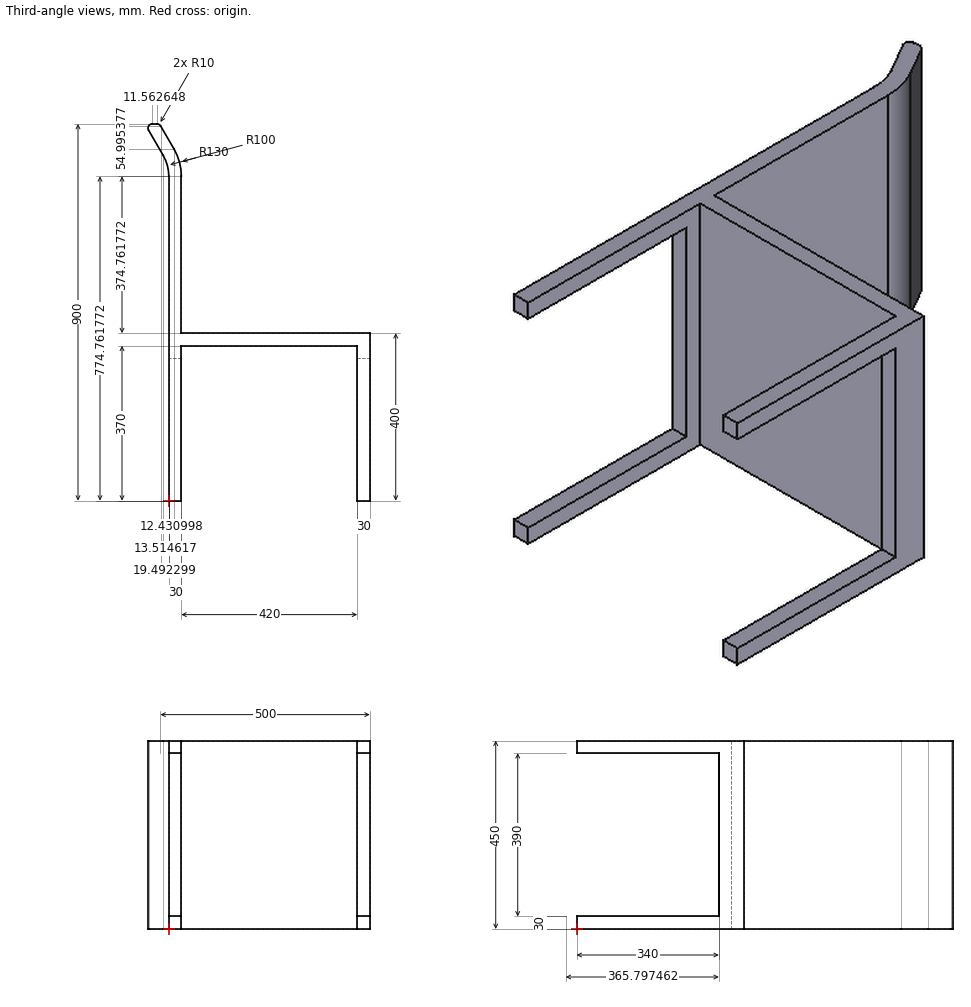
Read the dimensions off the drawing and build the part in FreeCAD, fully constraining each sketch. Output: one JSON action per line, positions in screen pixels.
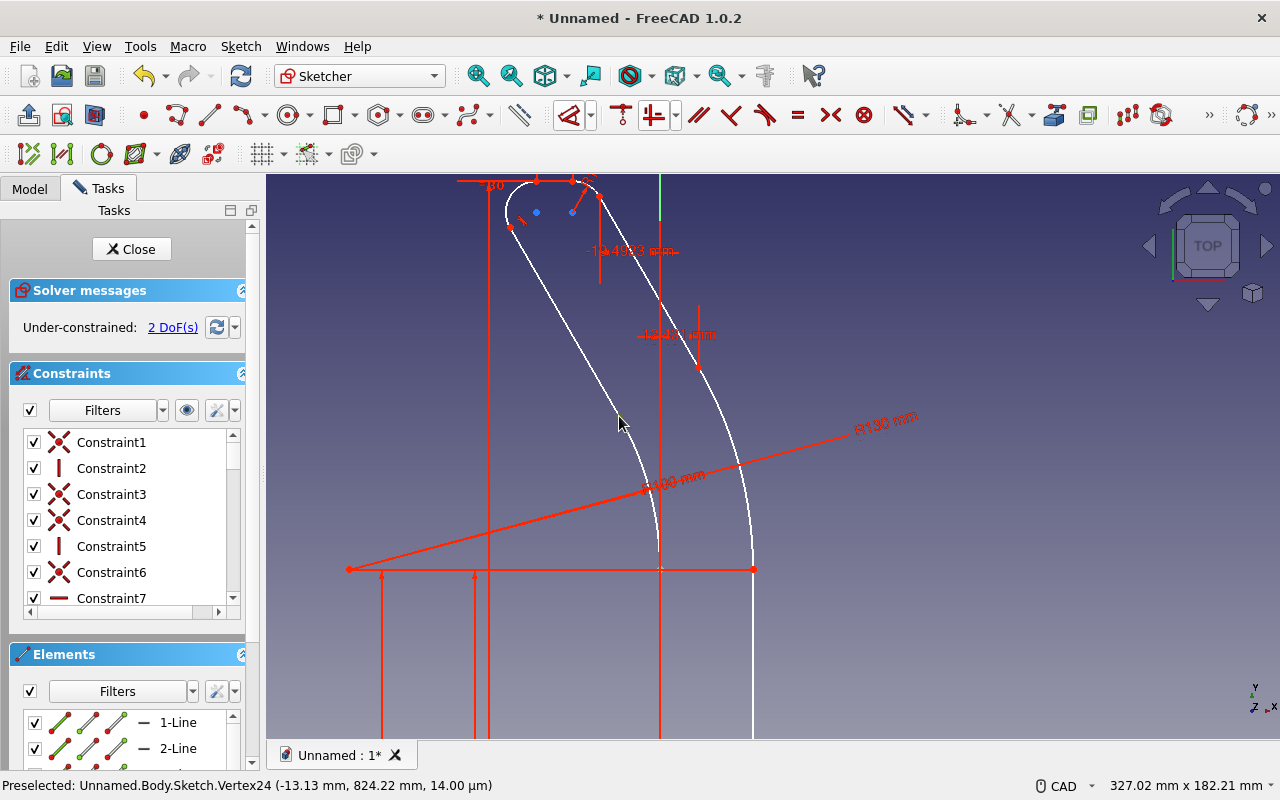
{"action": "left_click", "coordinate": [590, 116]}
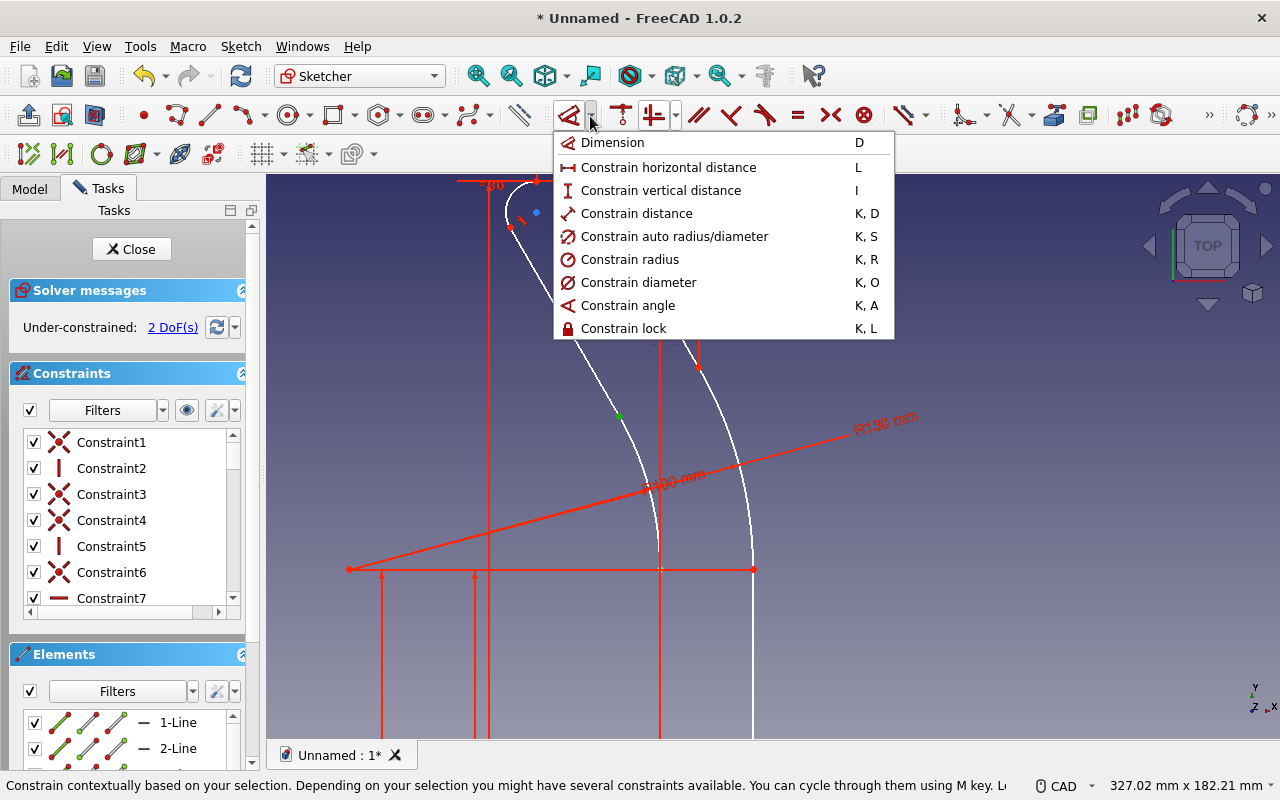
{"action": "left_click", "coordinate": [724, 168]}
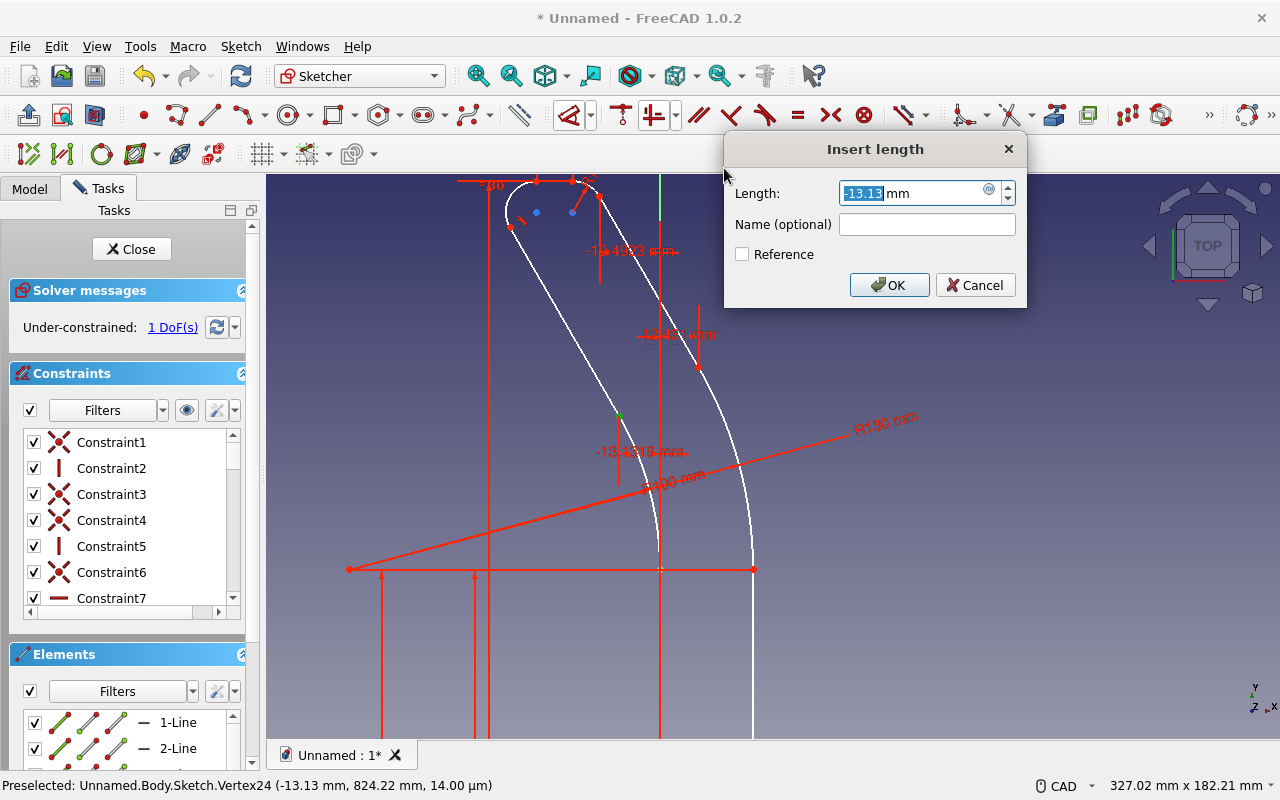
{"action": "type", "text": "-13.514617"}
{"action": "key", "text": "Return"}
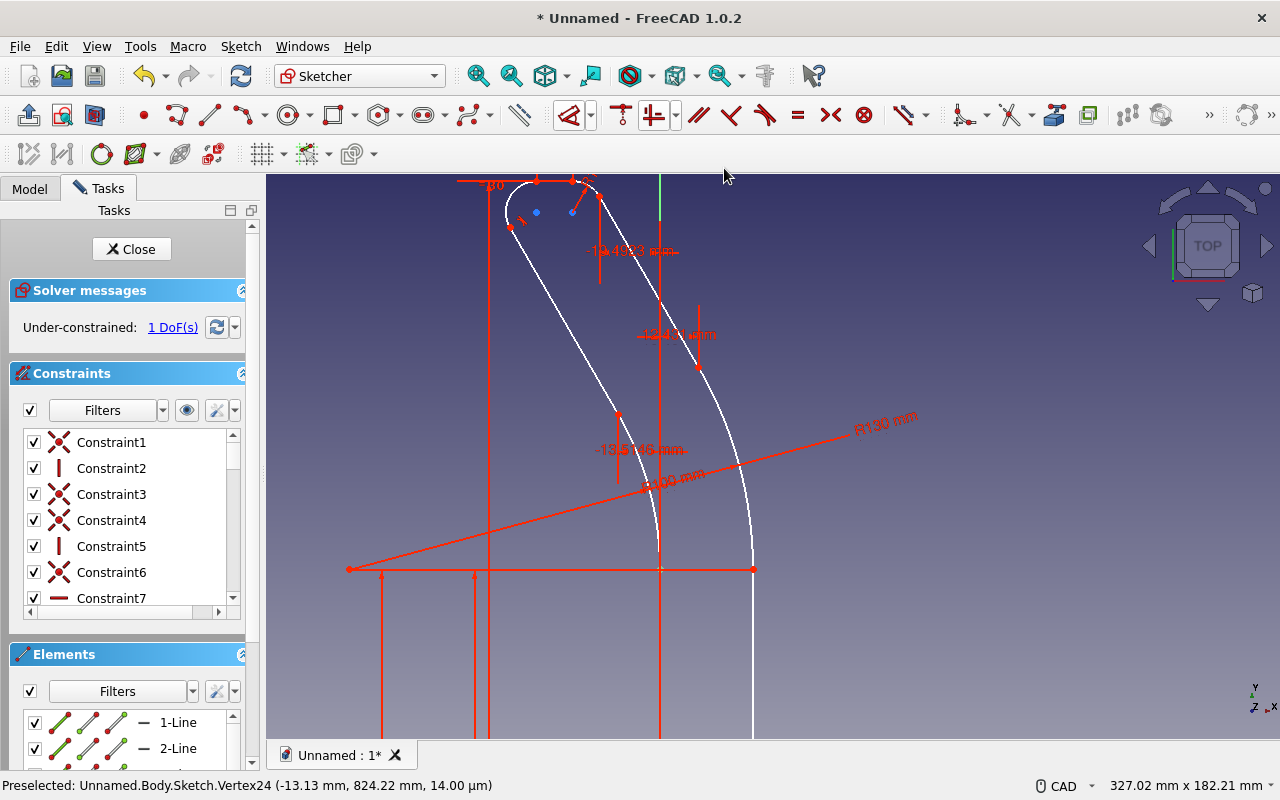
{"action": "left_click", "coordinate": [659, 299]}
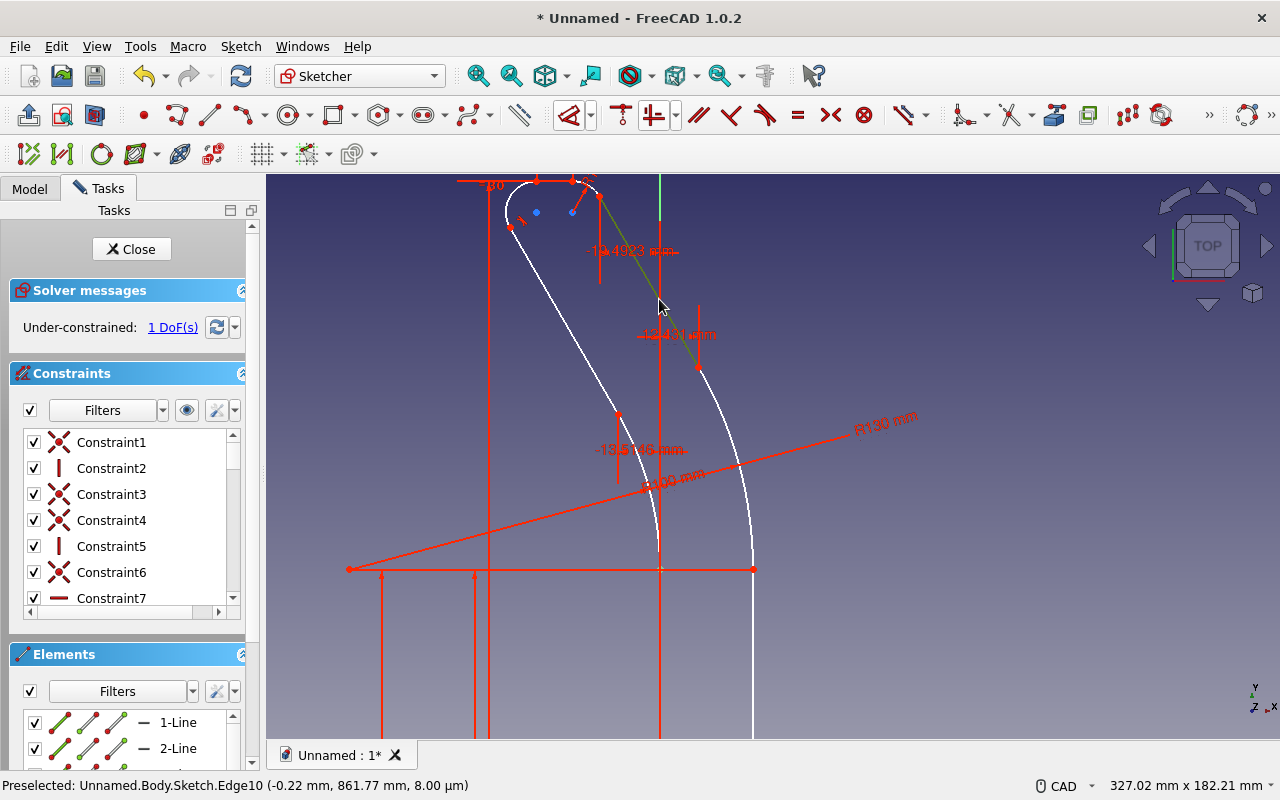
{"action": "key", "text": "i"}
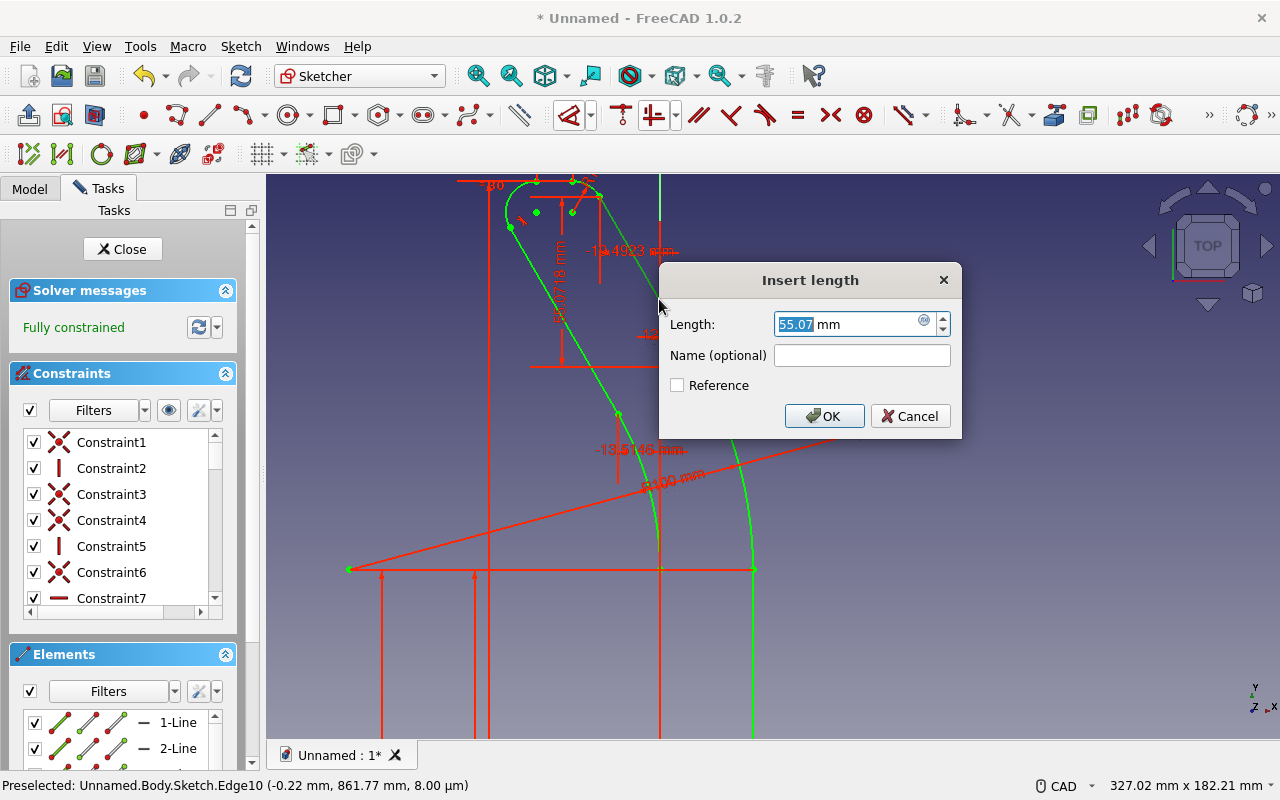
{"action": "type", "text": "54.995377"}
{"action": "key", "text": "Return"}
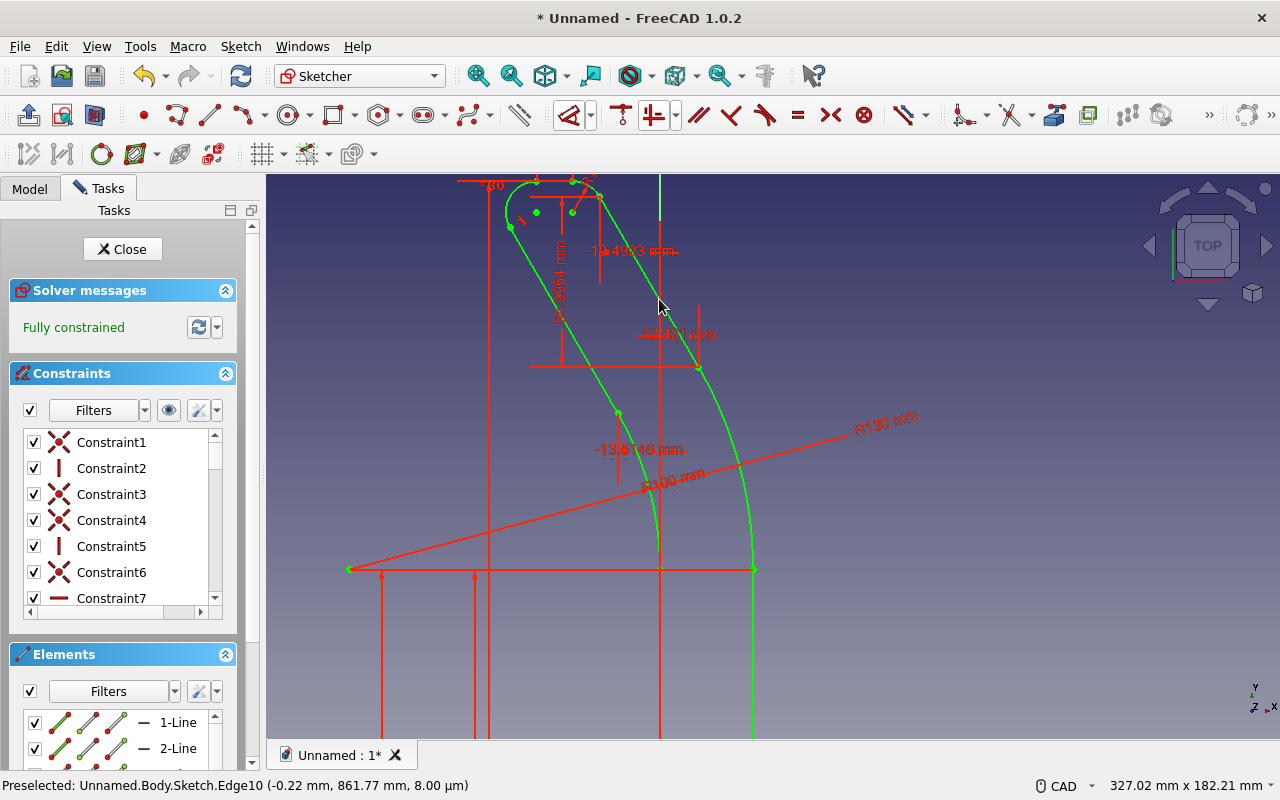
{"action": "left_click", "coordinate": [123, 249]}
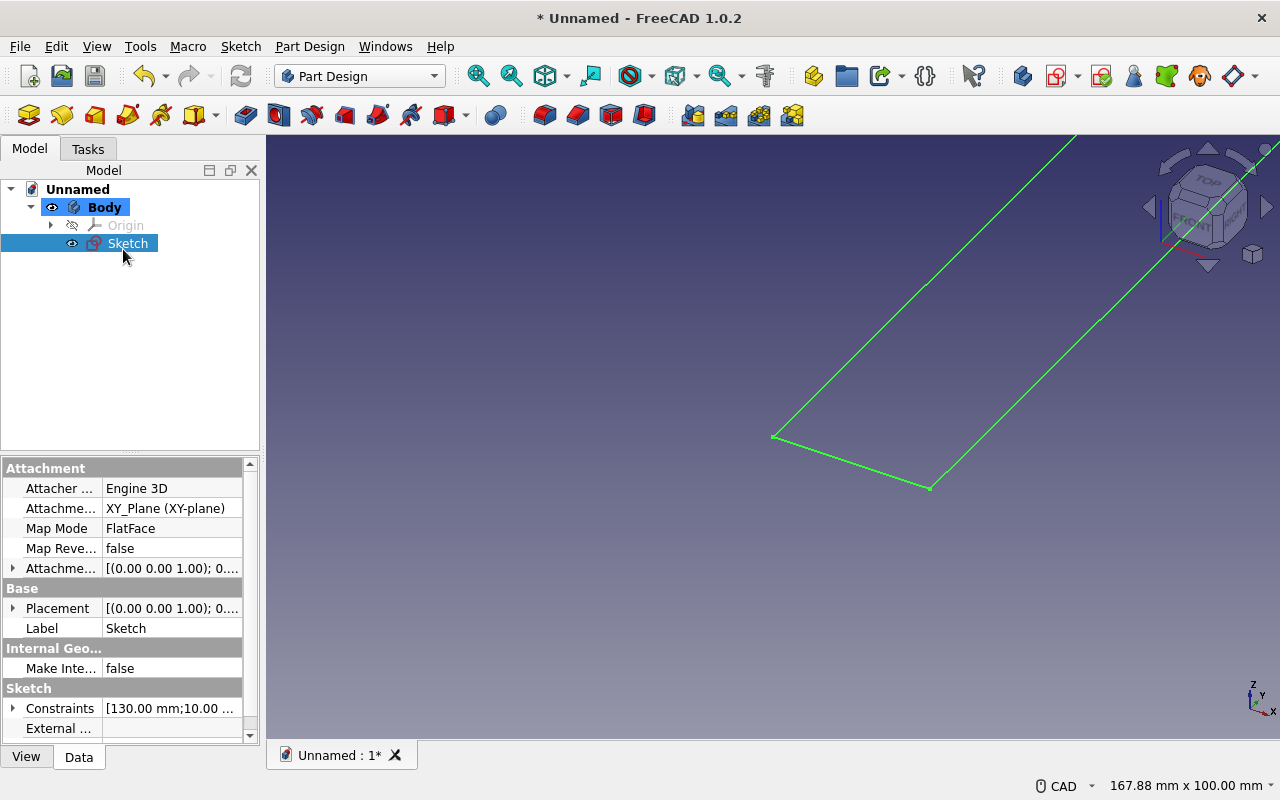
{"action": "left_click", "coordinate": [29, 116]}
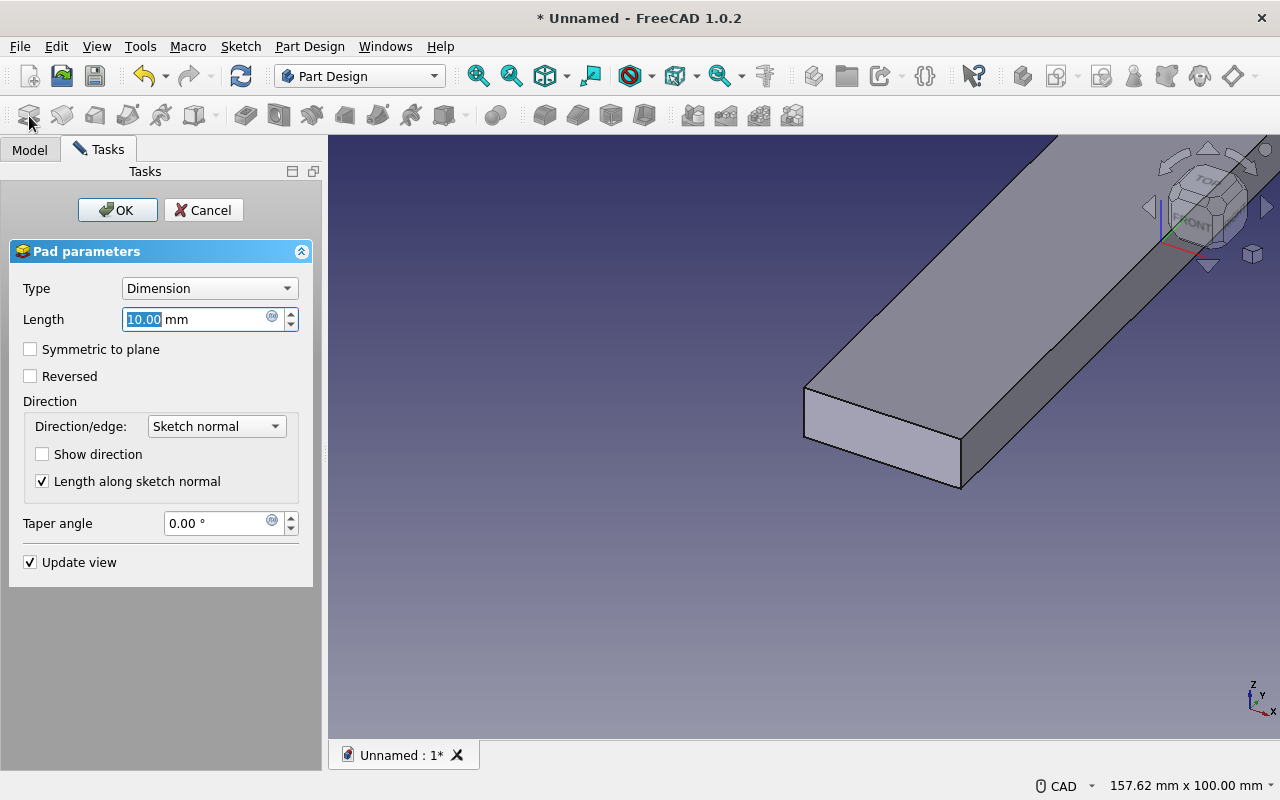
{"action": "type", "text": "450"}
{"action": "key", "text": "Tab"}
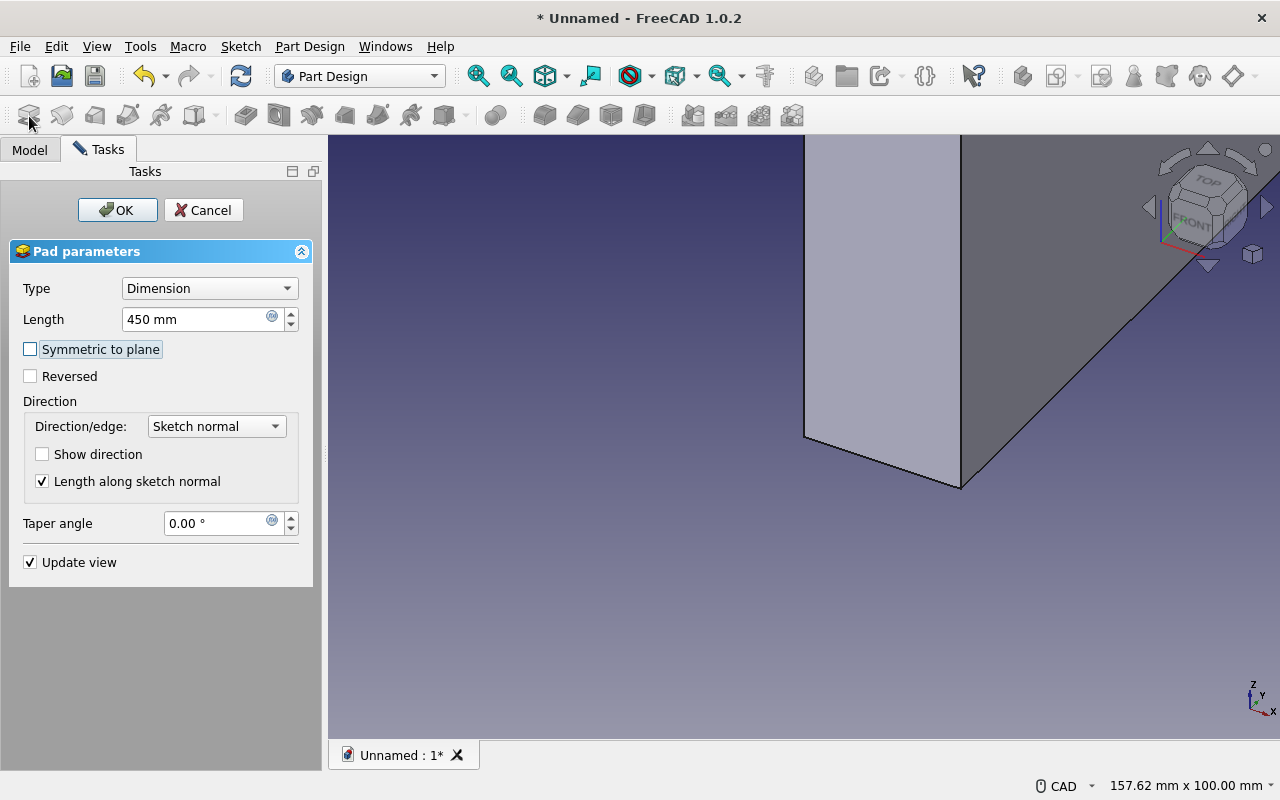
{"action": "left_click", "coordinate": [118, 210]}